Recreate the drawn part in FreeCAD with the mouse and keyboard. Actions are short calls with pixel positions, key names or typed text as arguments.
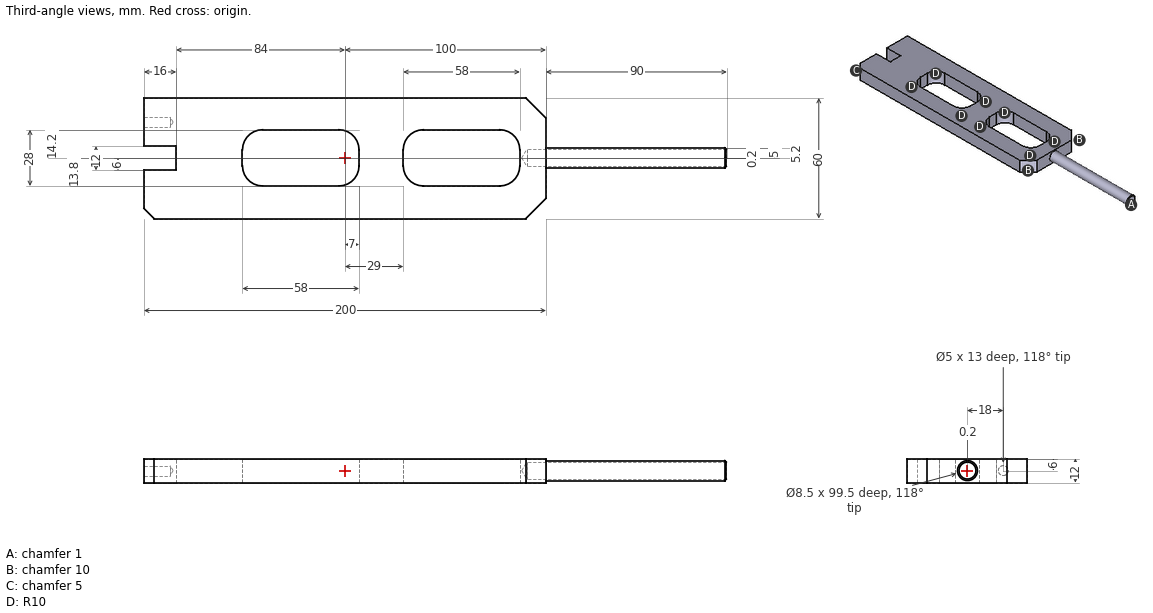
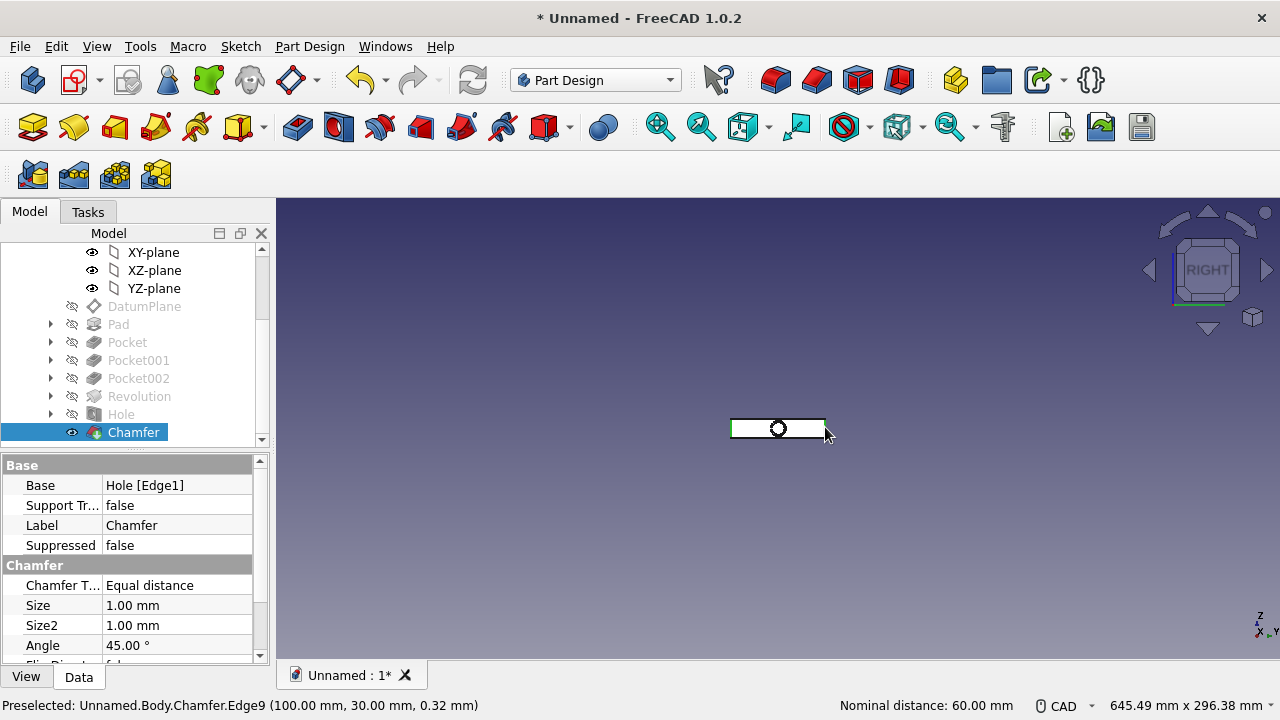
click(817, 80)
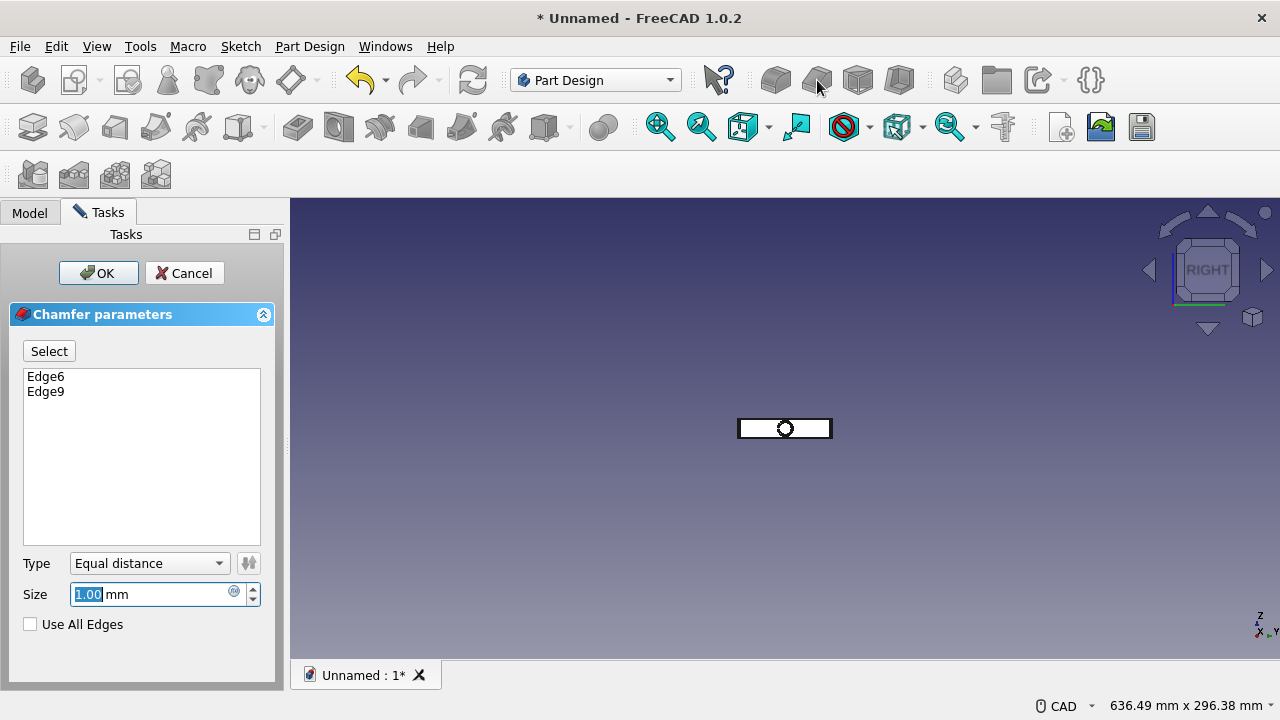
text(10)
key(Tab)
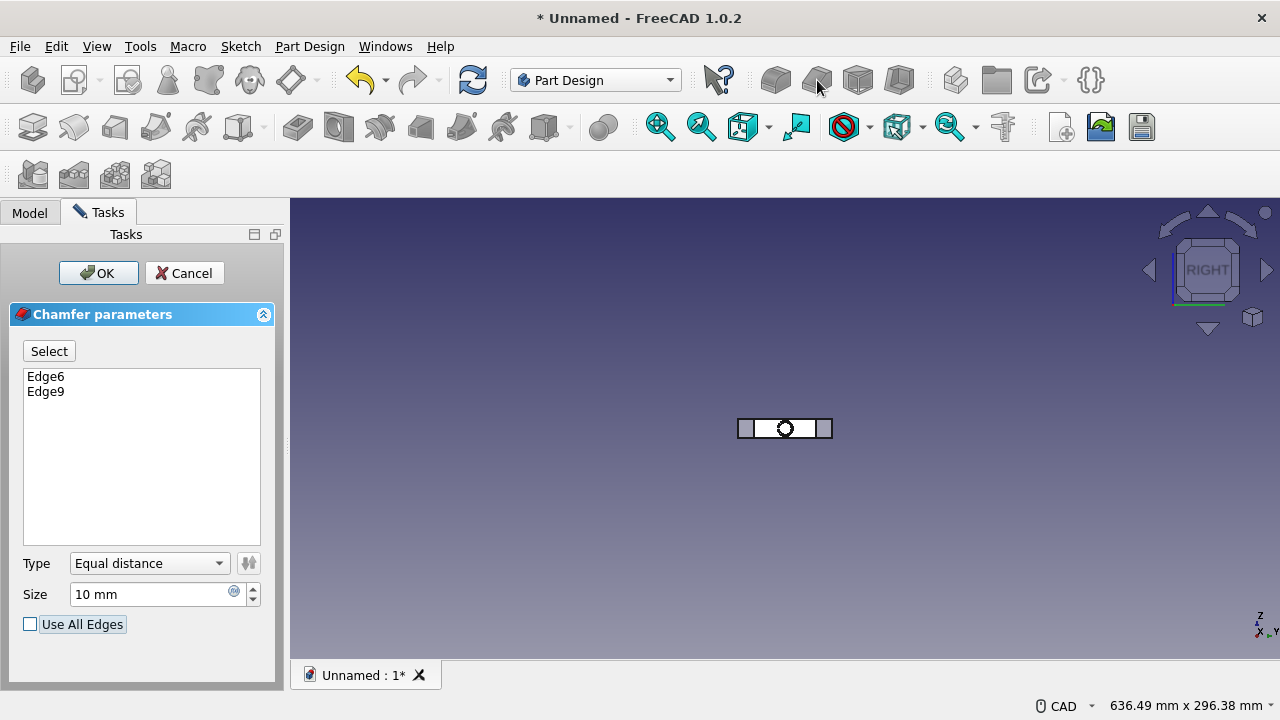
click(99, 273)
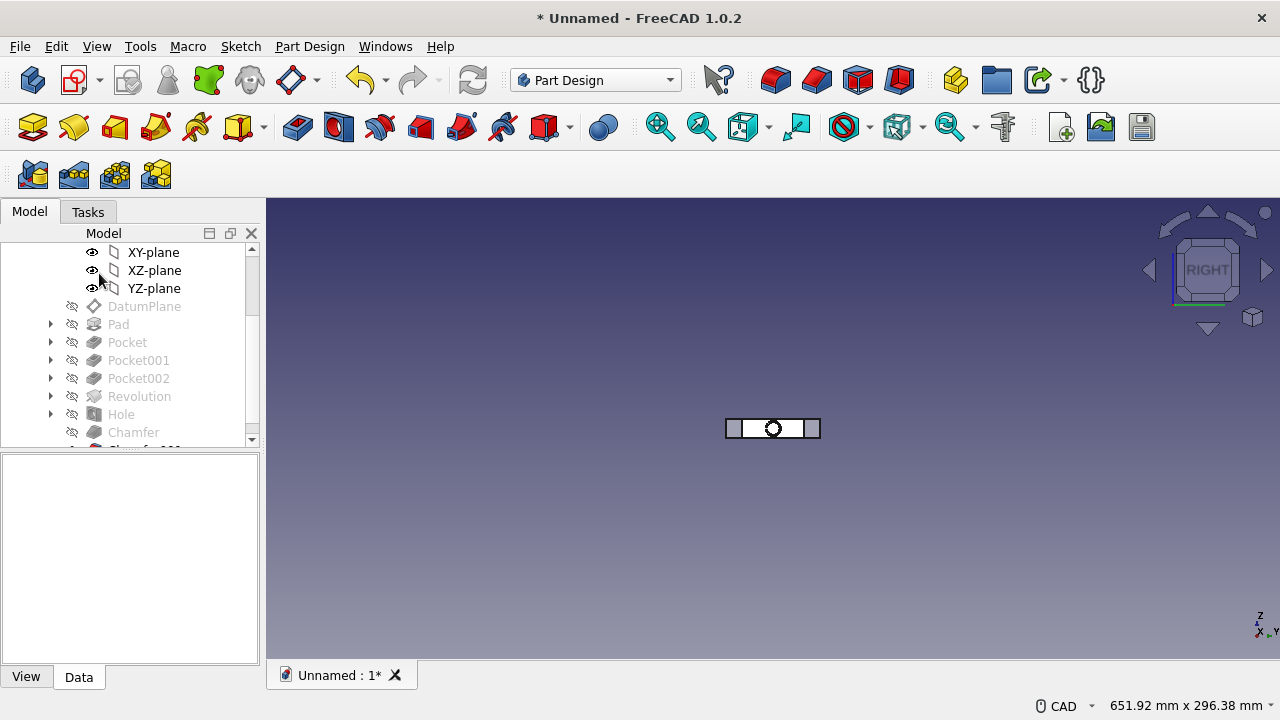
click(661, 128)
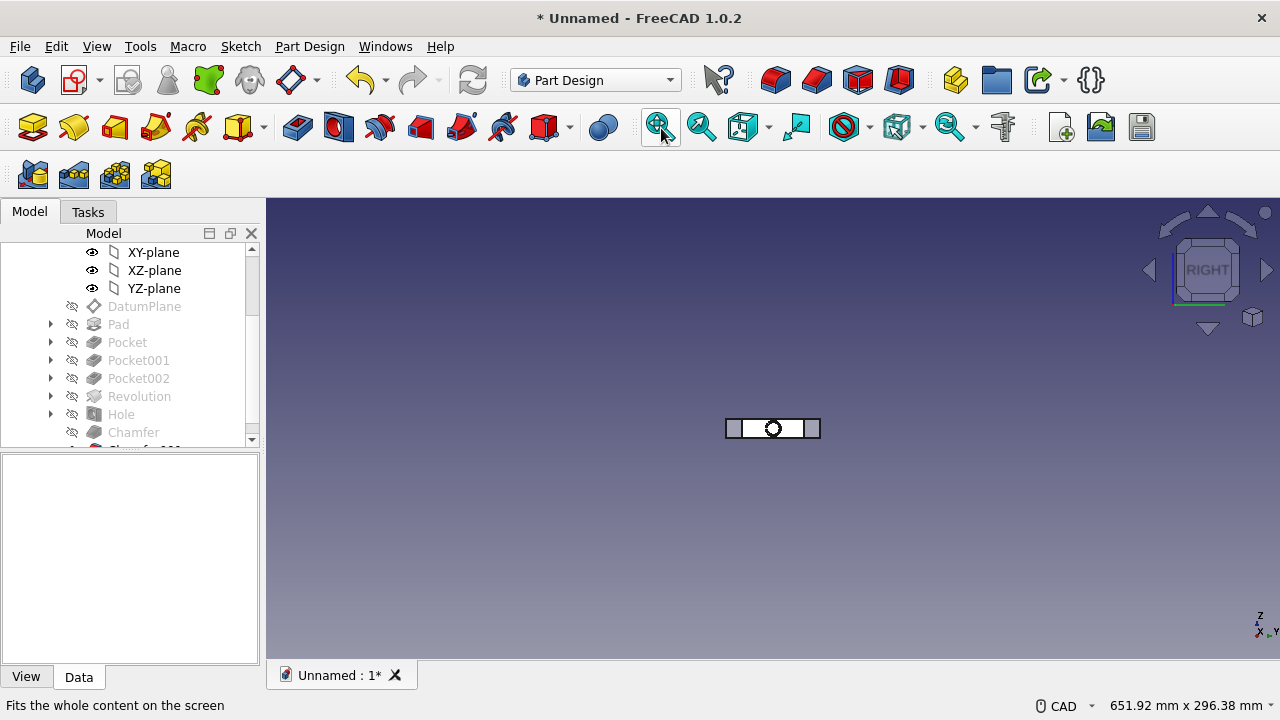
scroll(726, 427, up, 4)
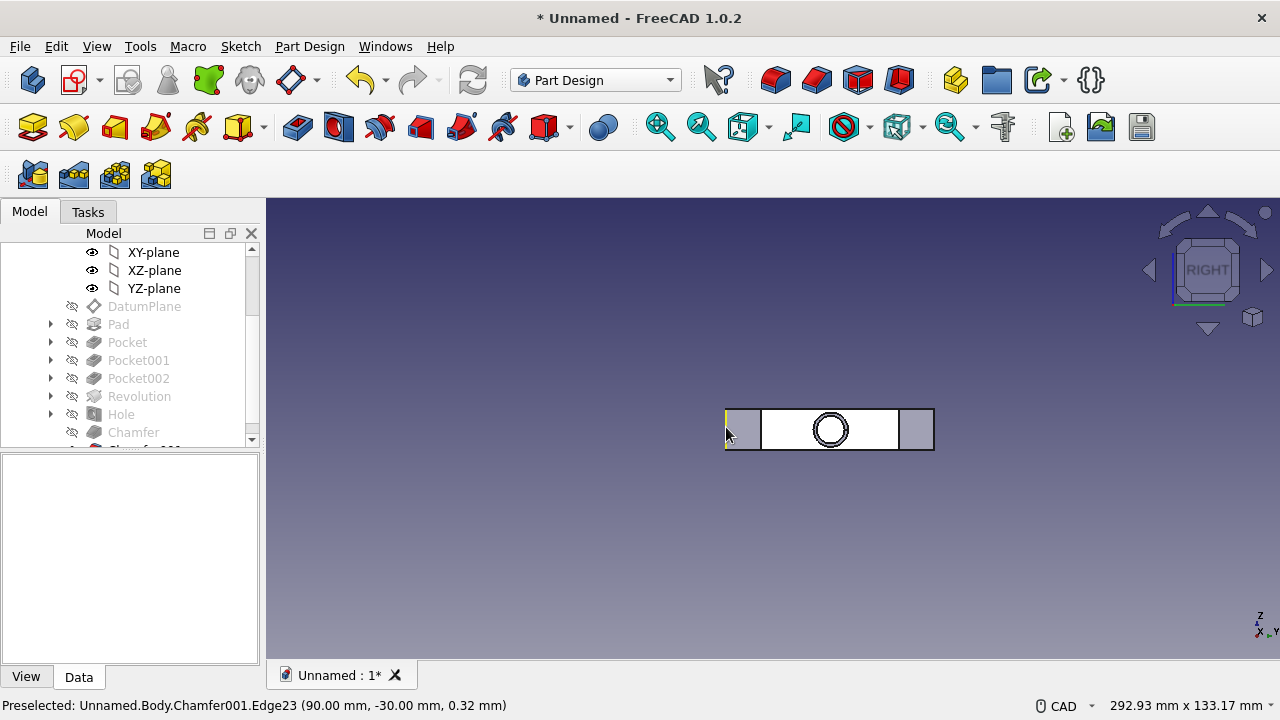
key(v)
key(f)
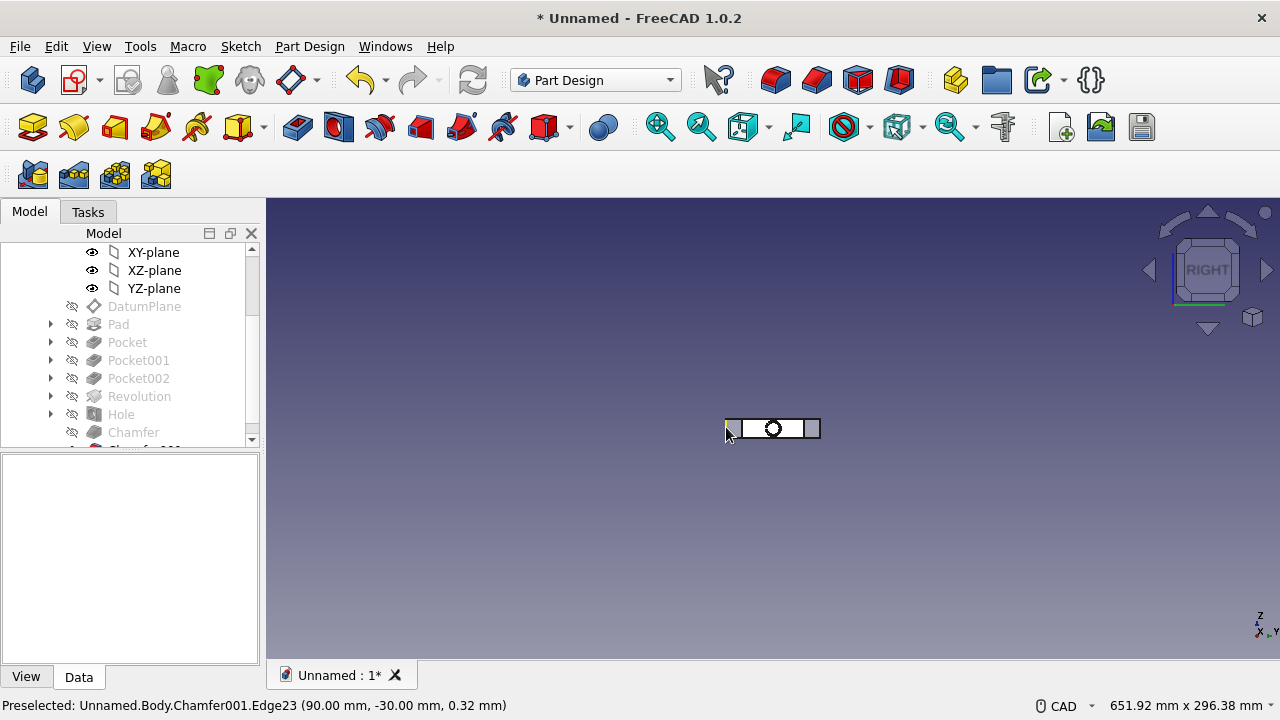
key(0)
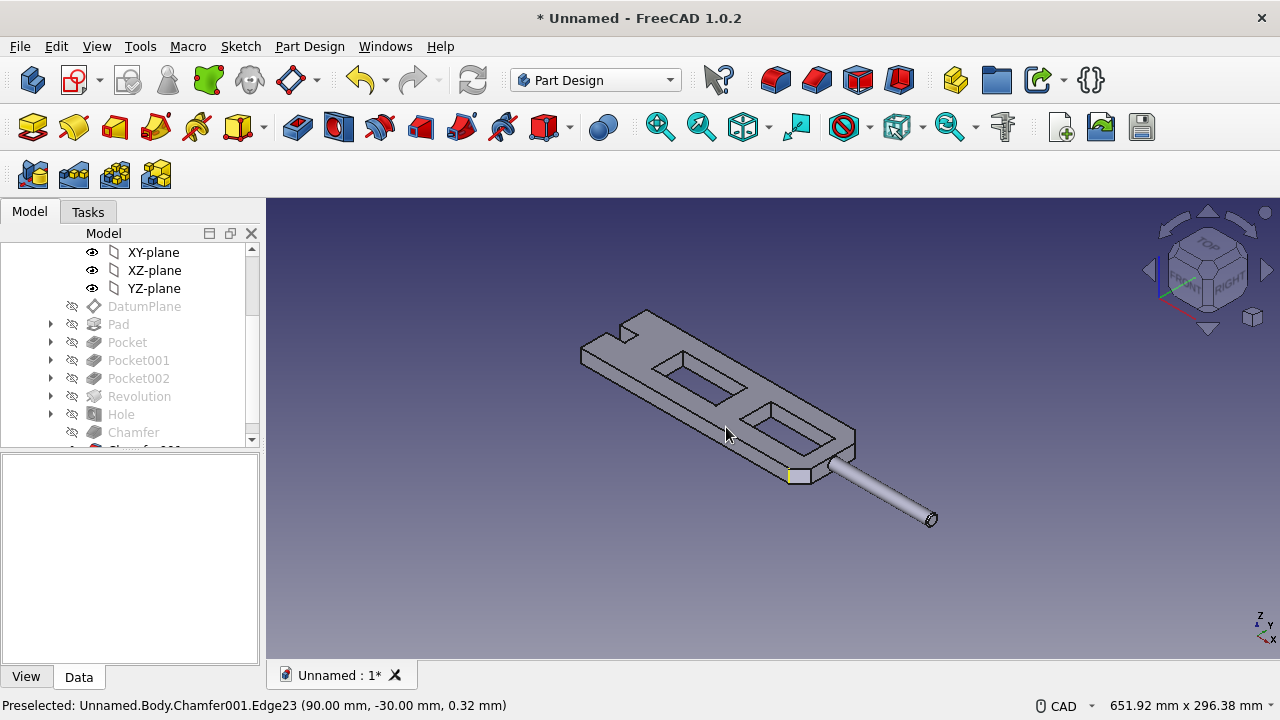
scroll(581, 354, up, 4)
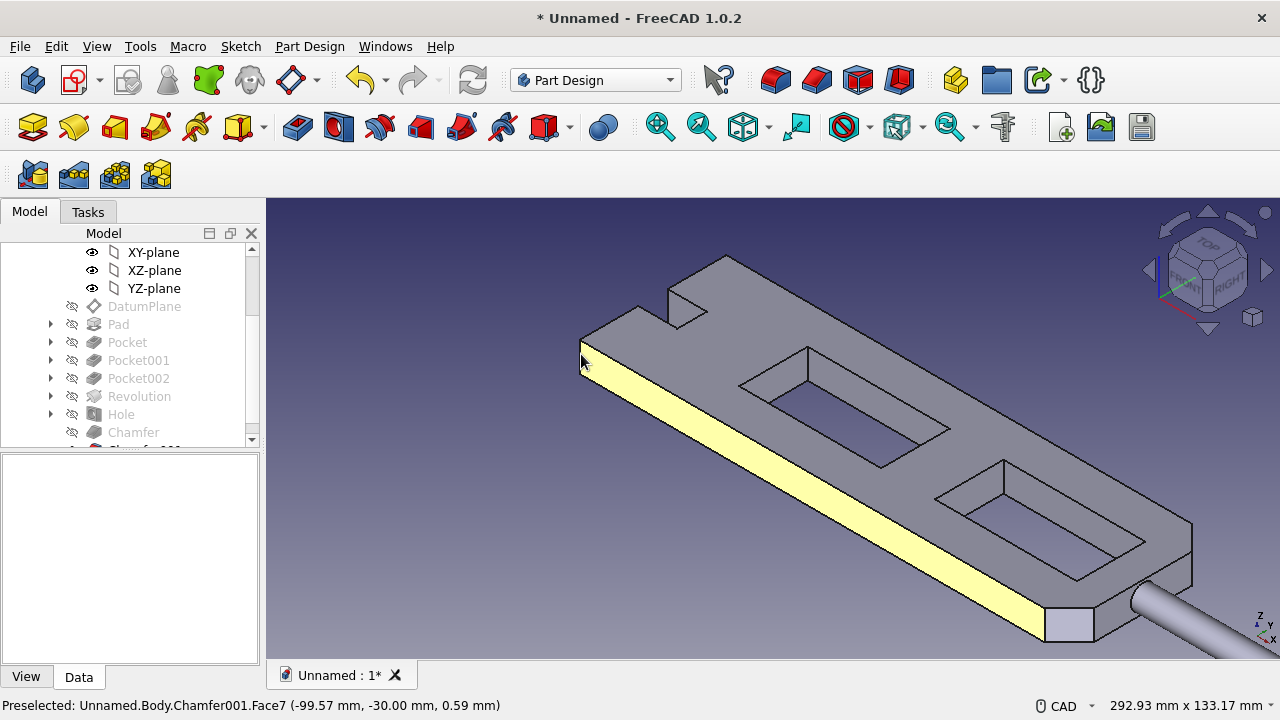
key(v)
key(f)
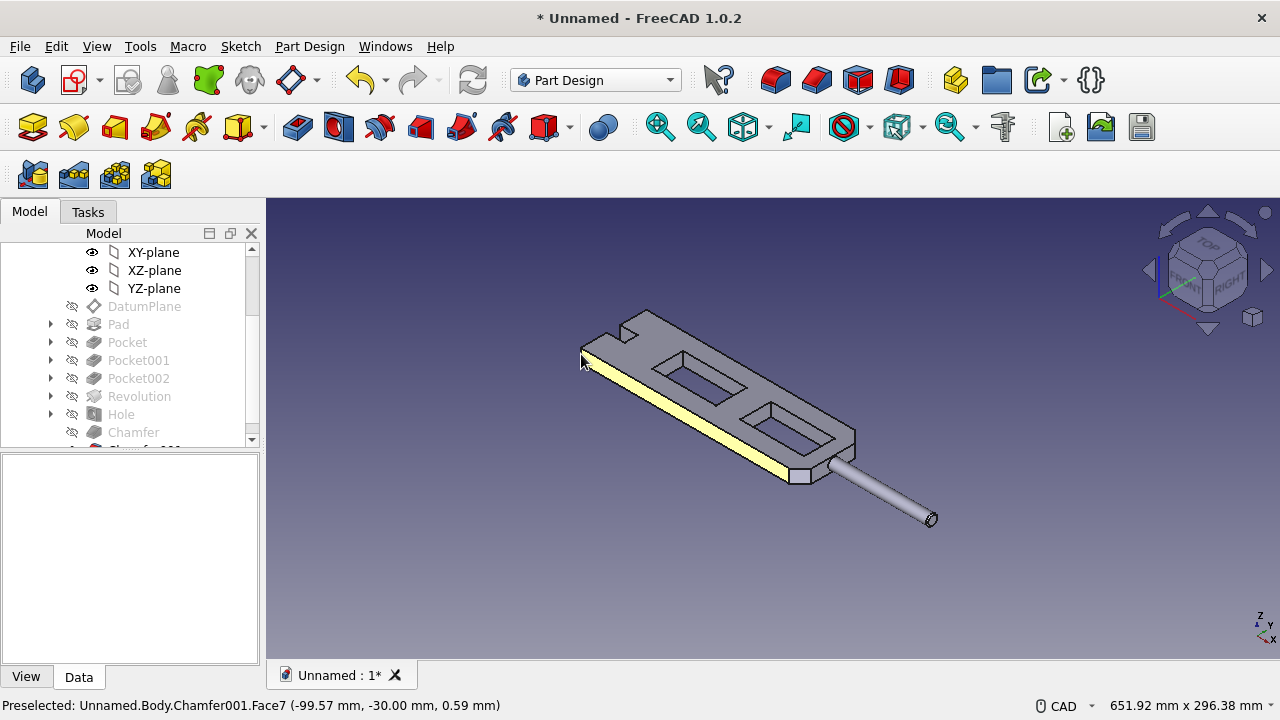
key(2)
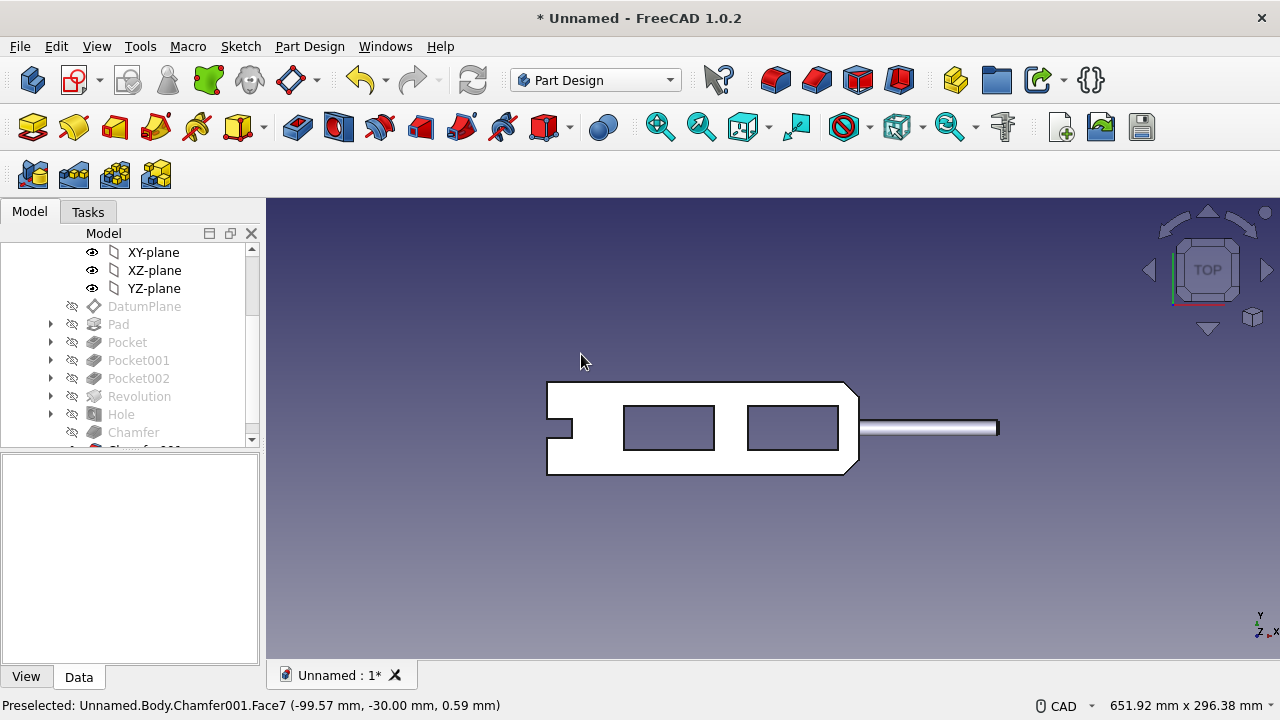
key(v)
key(f)